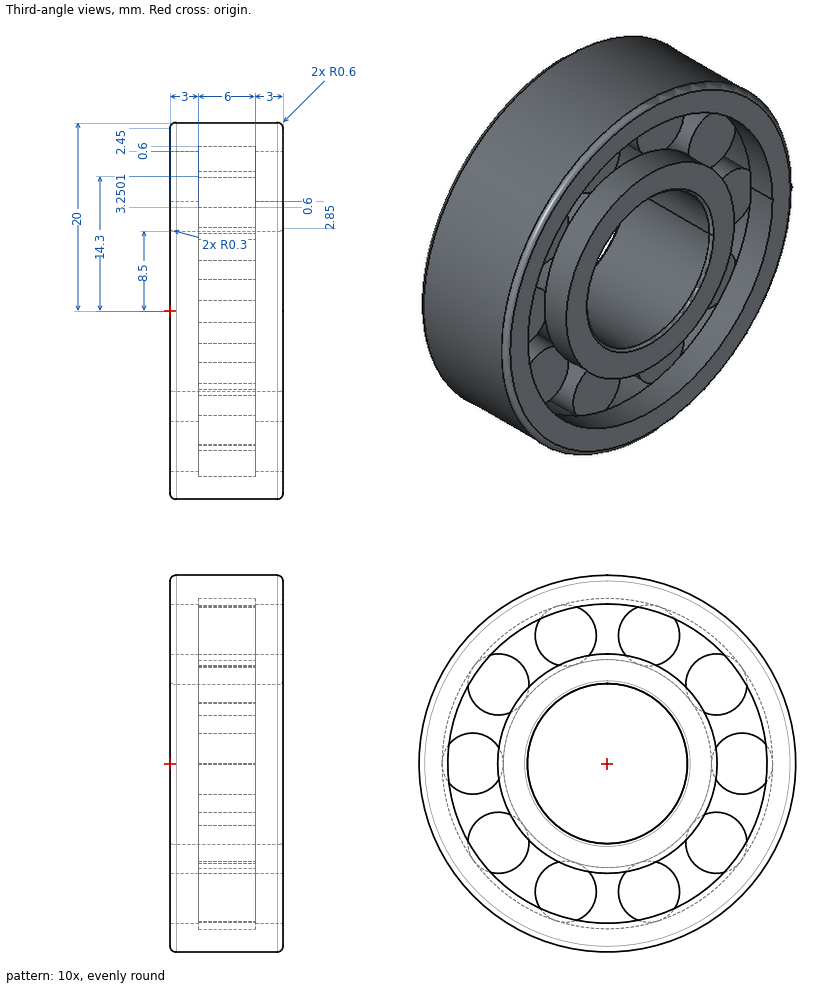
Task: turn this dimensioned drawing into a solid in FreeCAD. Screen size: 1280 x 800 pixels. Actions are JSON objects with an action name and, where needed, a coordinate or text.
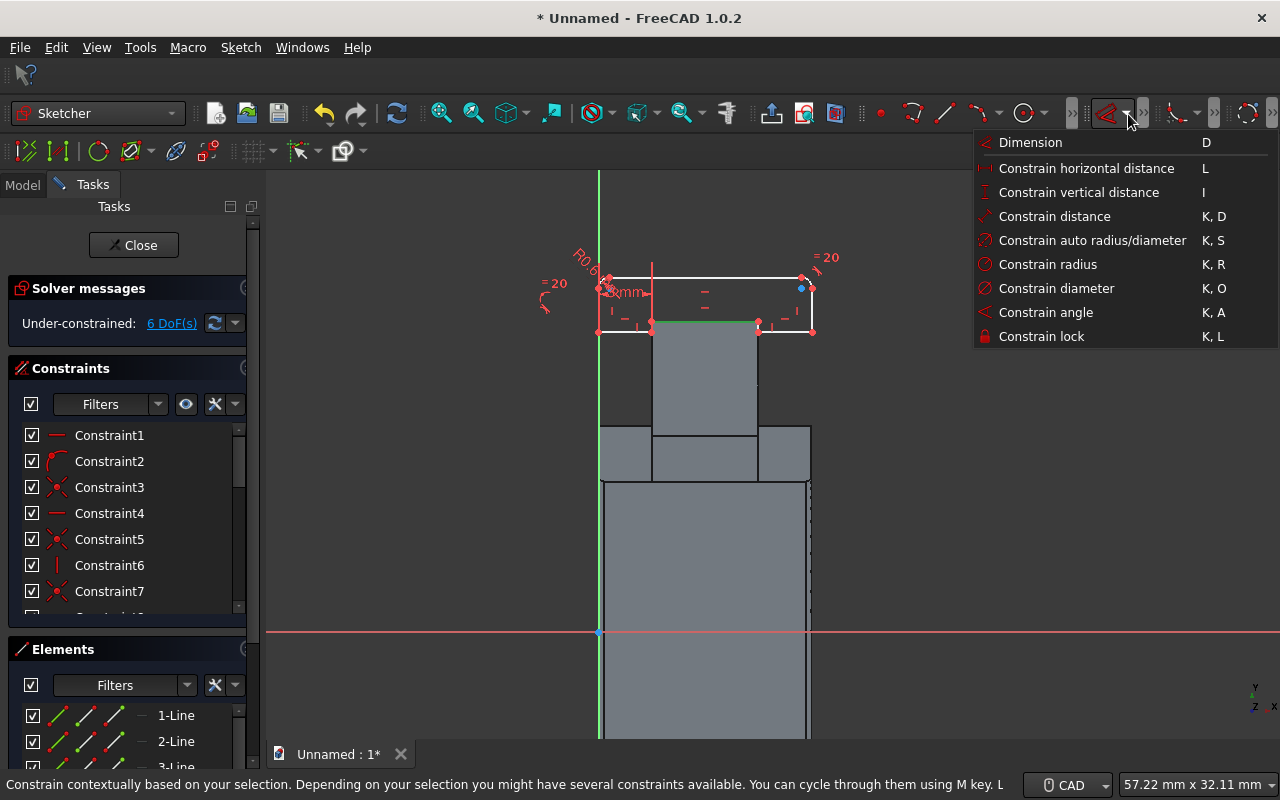
{"action": "left_click", "coordinate": [1126, 168]}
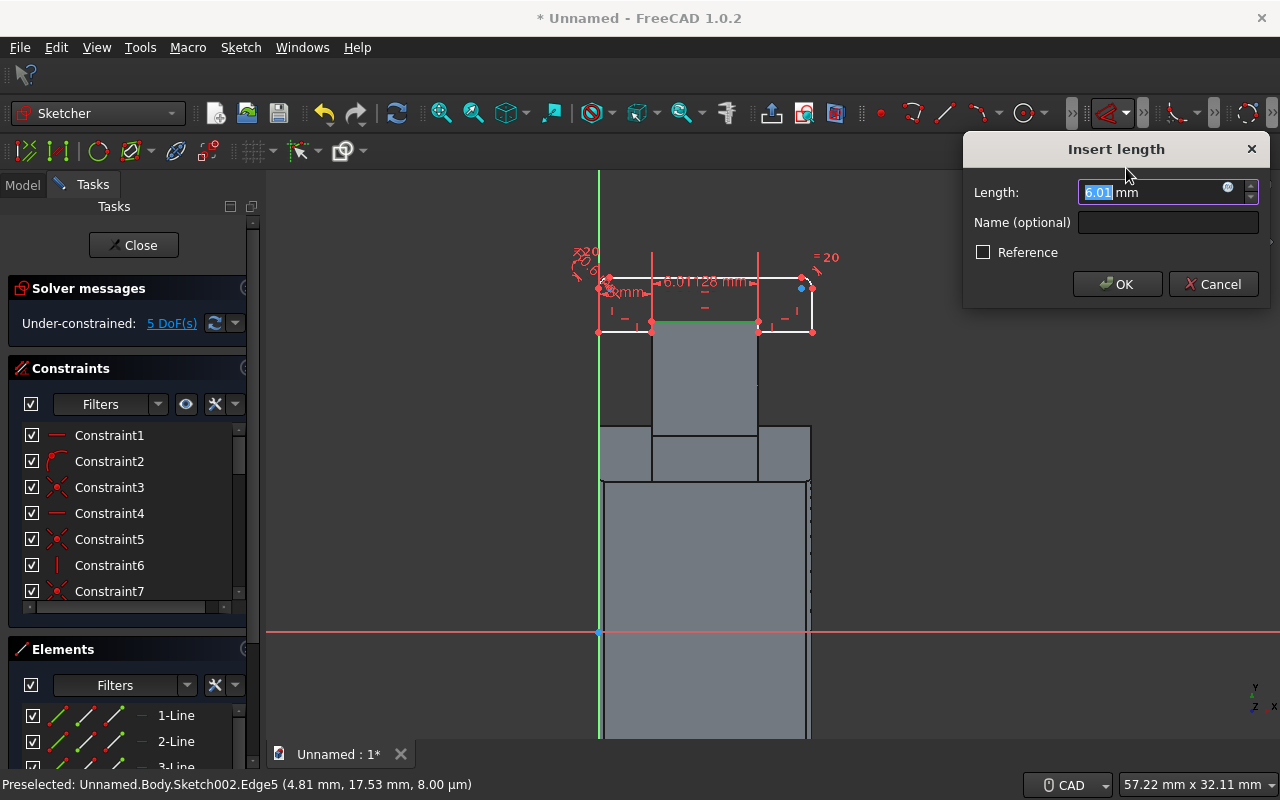
{"action": "type", "text": "6"}
{"action": "key", "text": "Return"}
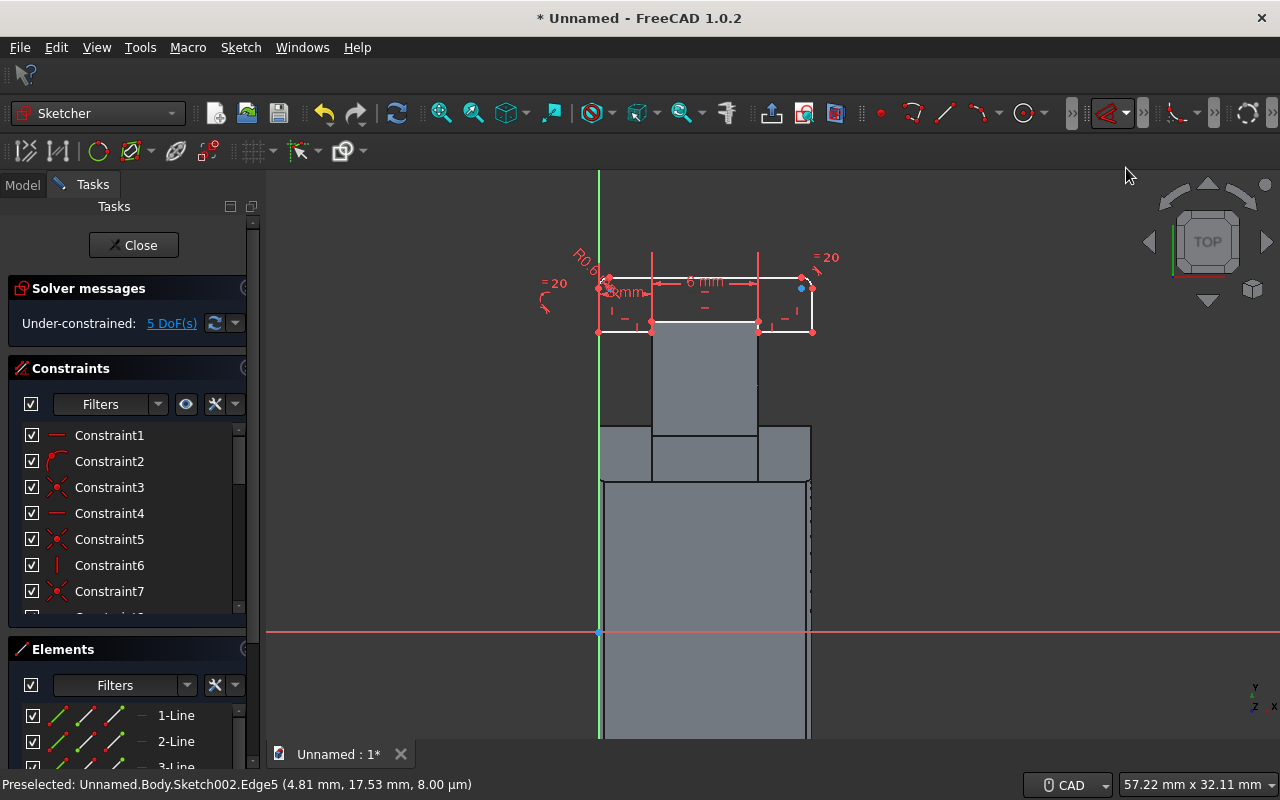
{"action": "left_click", "coordinate": [774, 332]}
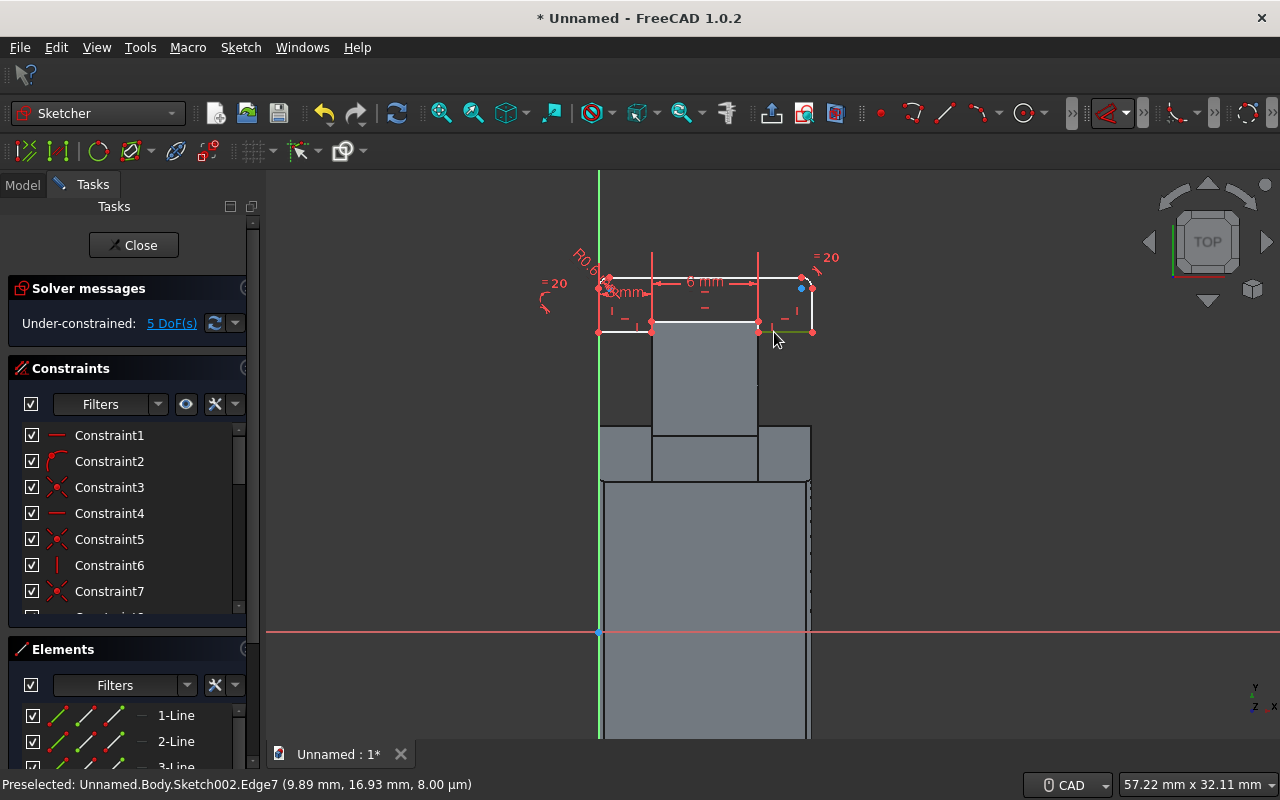
{"action": "left_click", "coordinate": [1128, 114]}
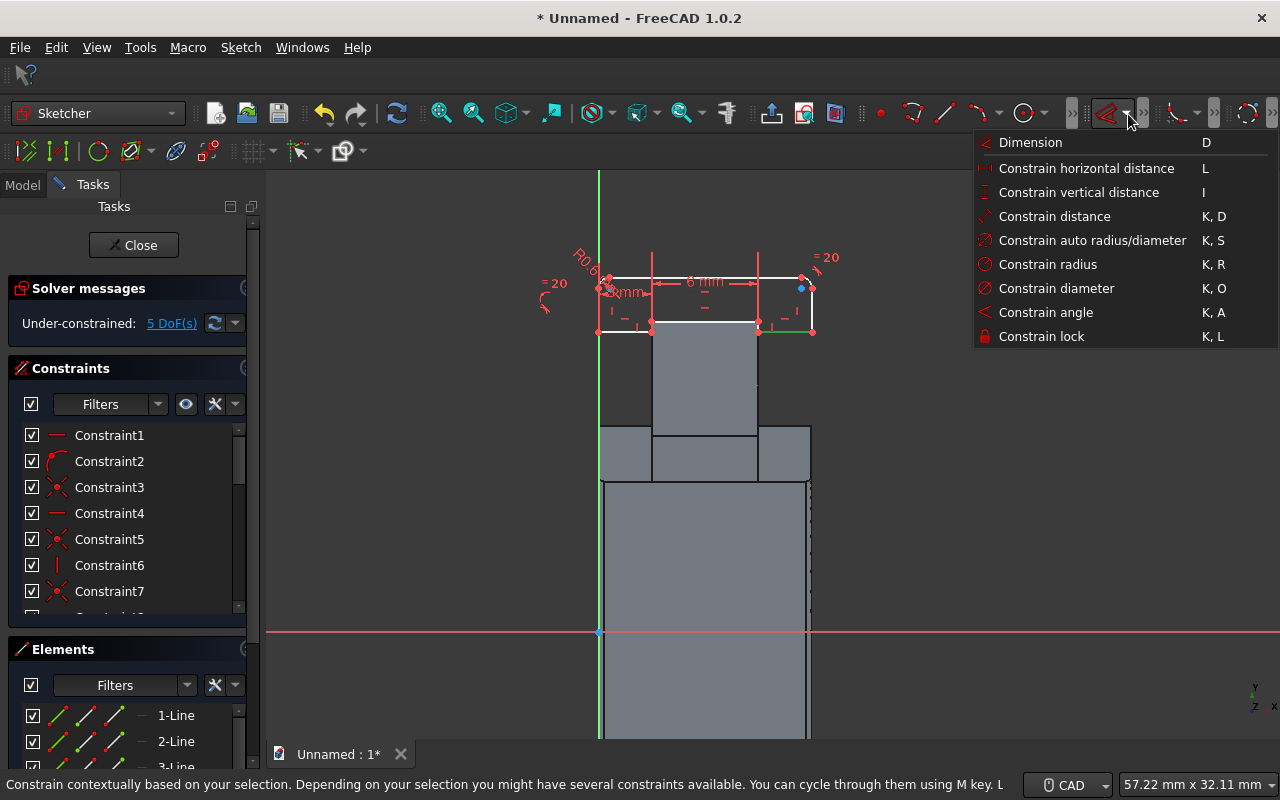
{"action": "left_click", "coordinate": [1126, 168]}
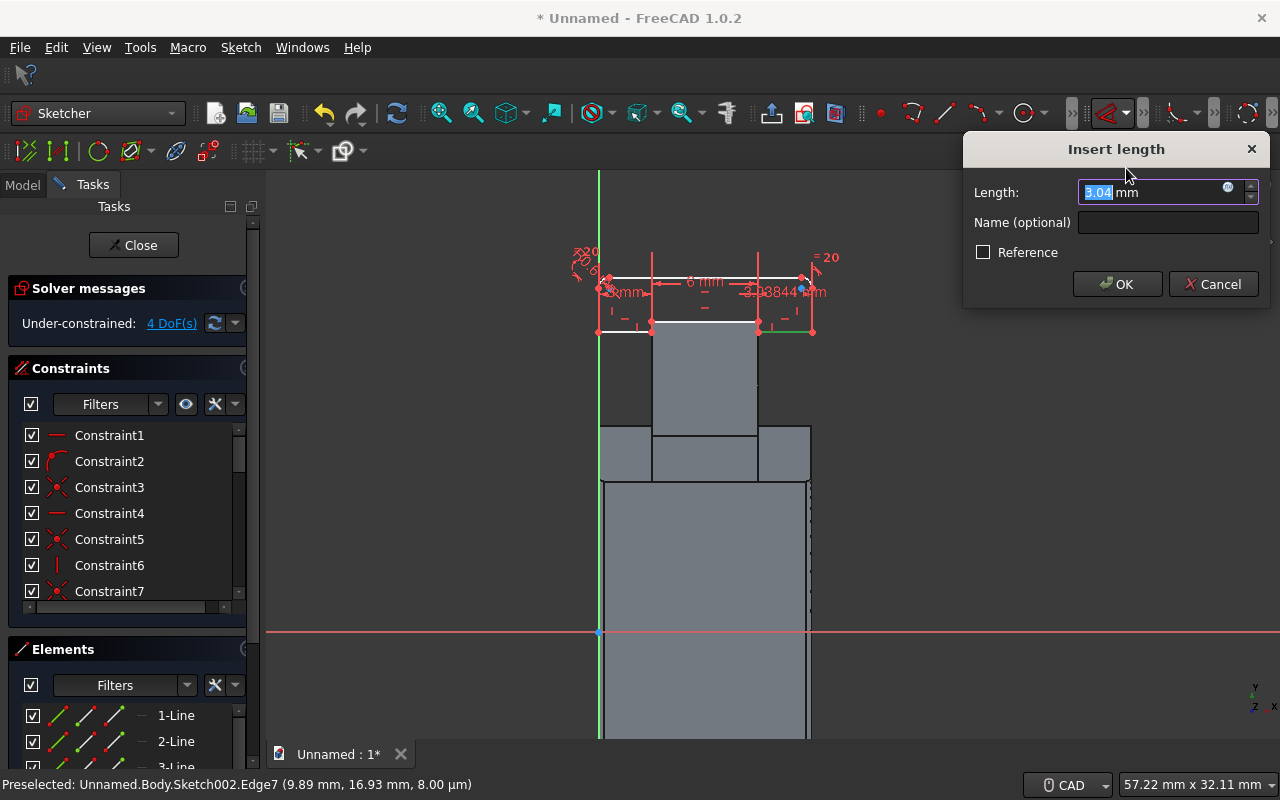
{"action": "type", "text": "3"}
{"action": "key", "text": "Return"}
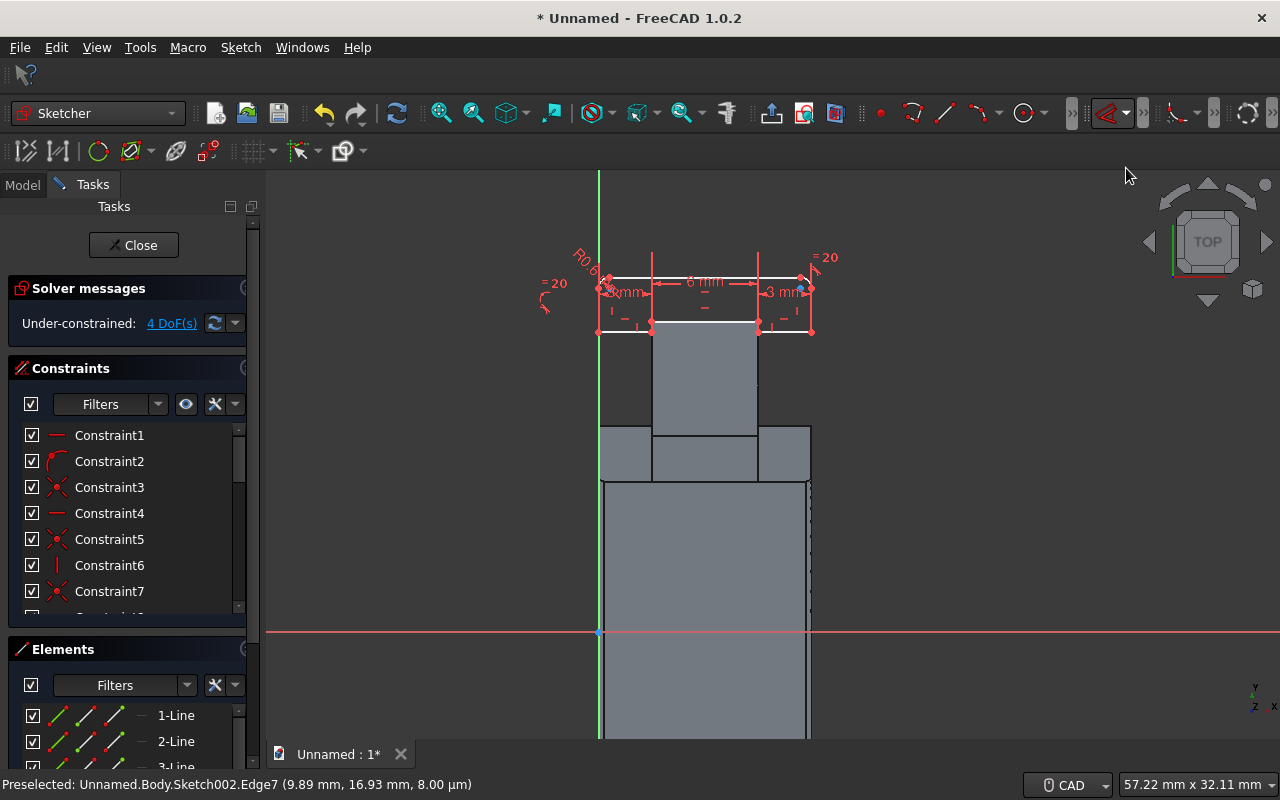
{"action": "scroll", "coordinate": [652, 327], "scroll_direction": "up", "scroll_amount": 7}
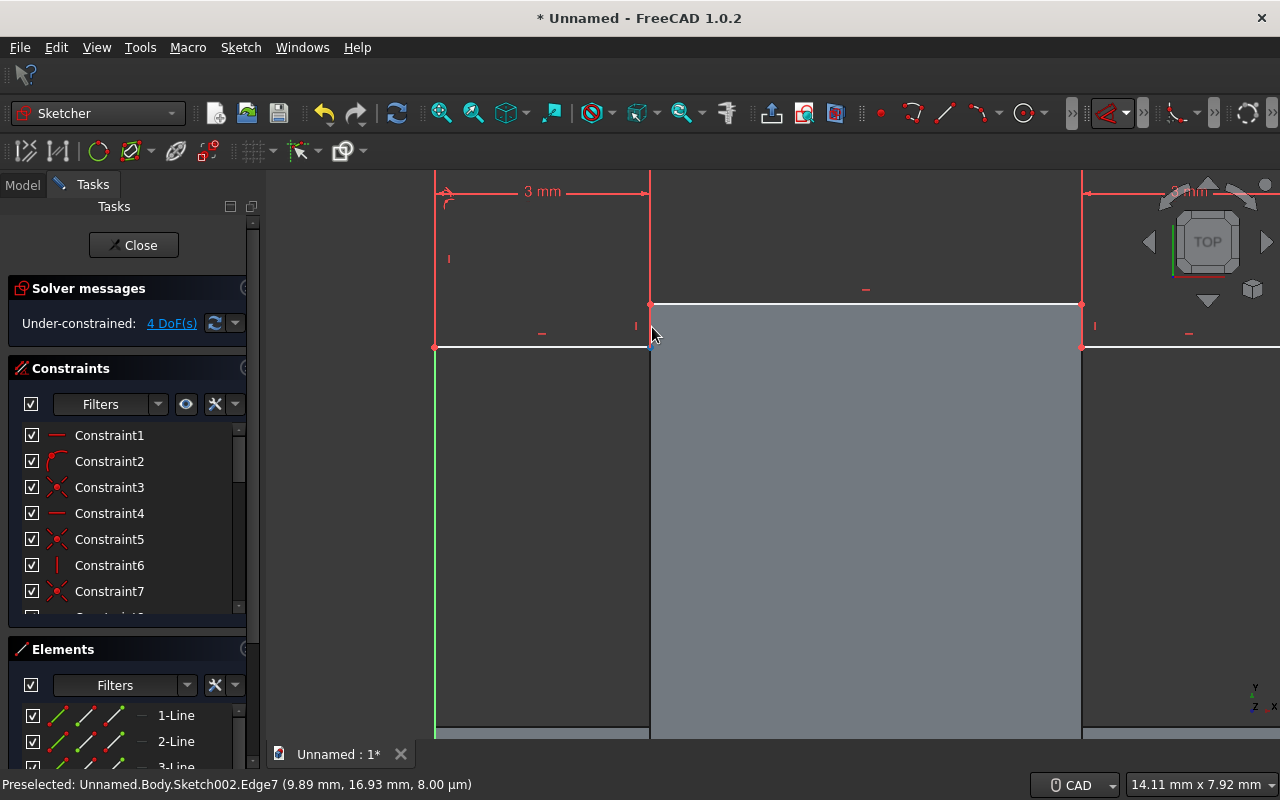
{"action": "left_click", "coordinate": [650, 326]}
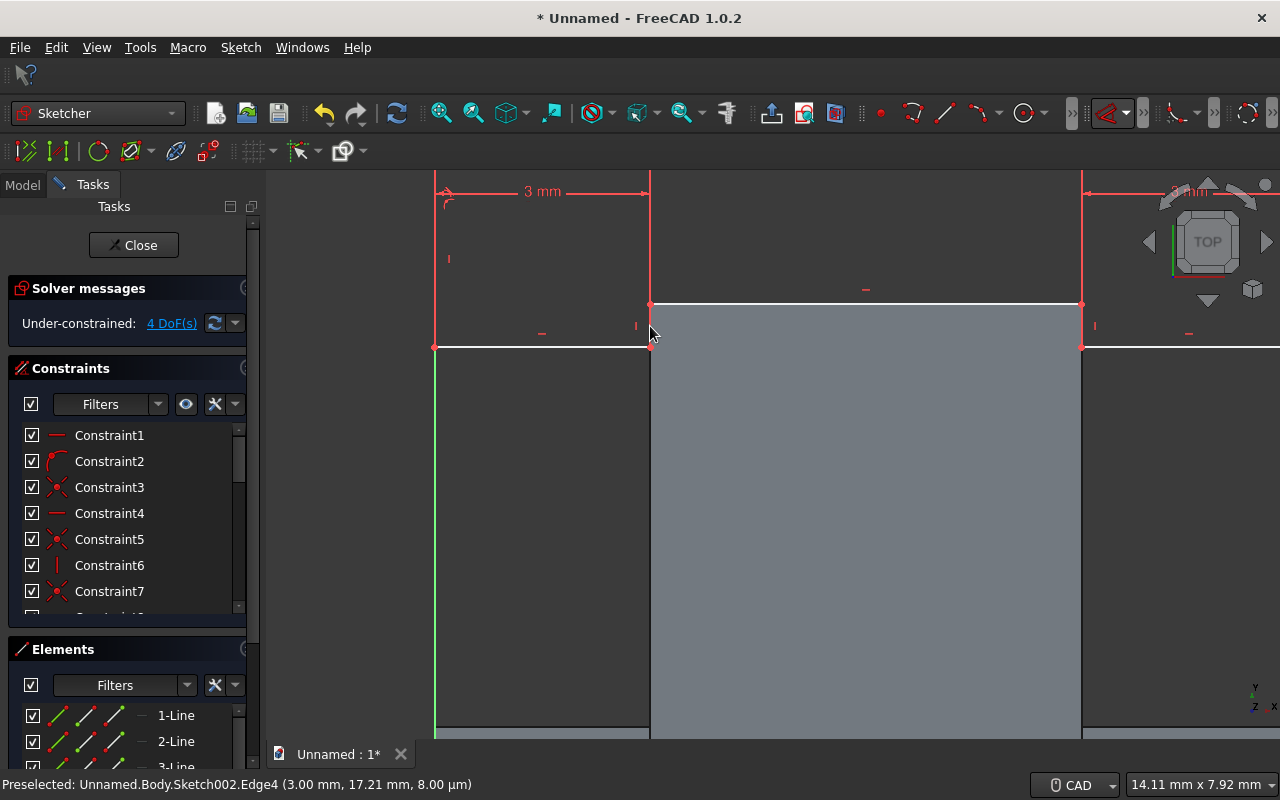
{"action": "key", "text": "i"}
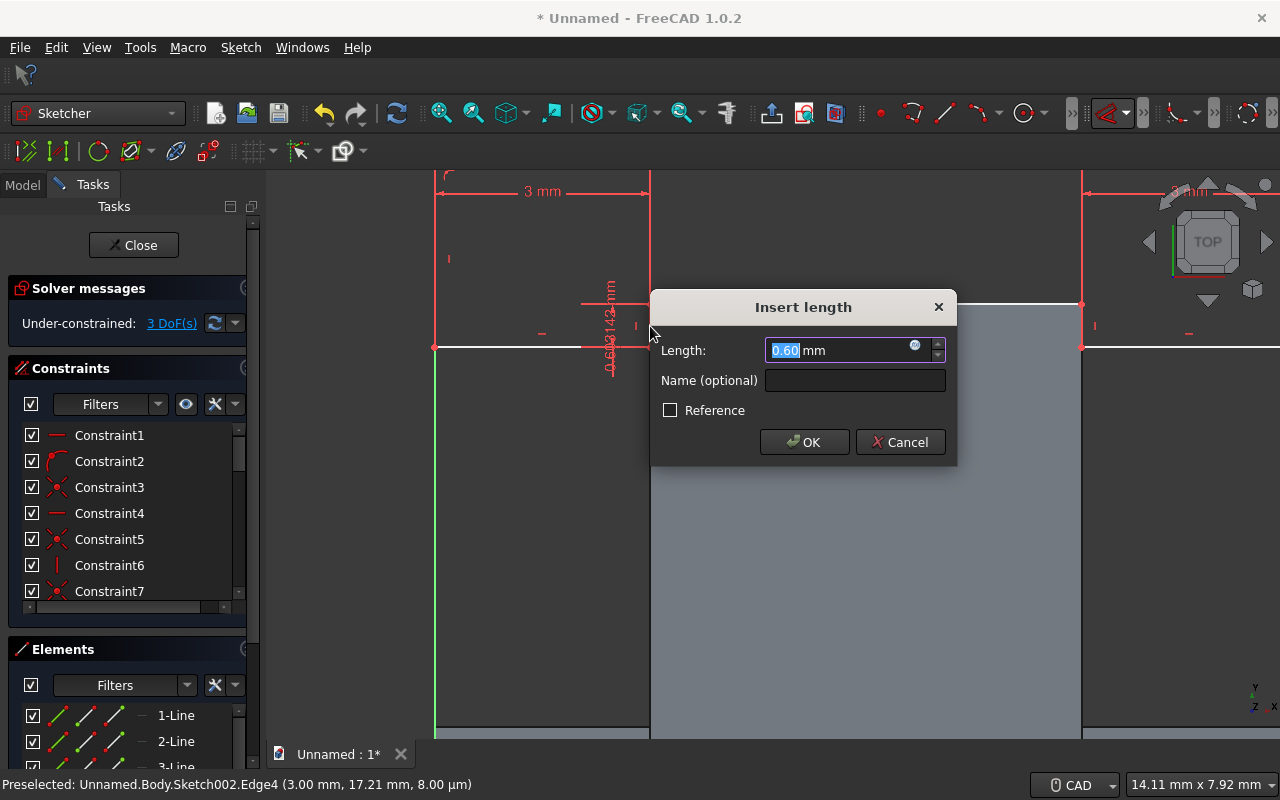
{"action": "type", "text": "0.6"}
{"action": "key", "text": "Return"}